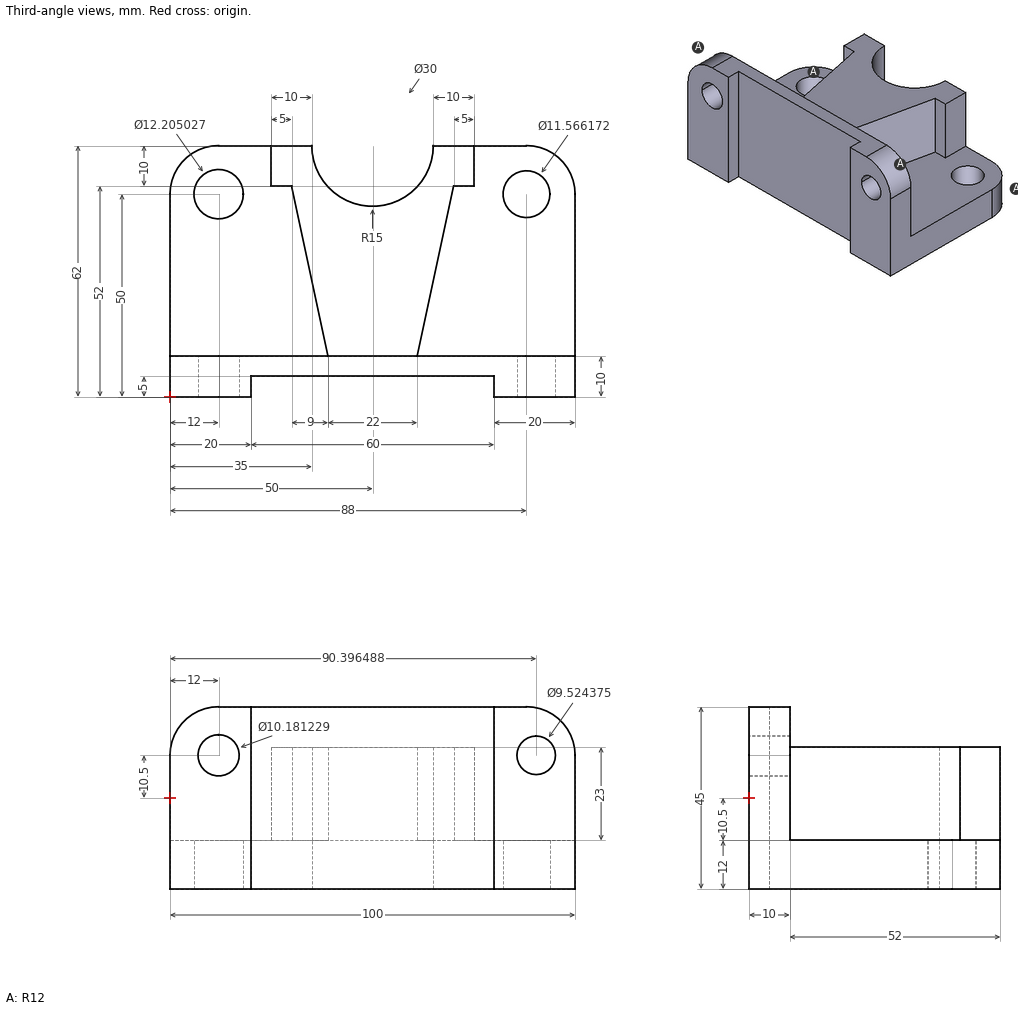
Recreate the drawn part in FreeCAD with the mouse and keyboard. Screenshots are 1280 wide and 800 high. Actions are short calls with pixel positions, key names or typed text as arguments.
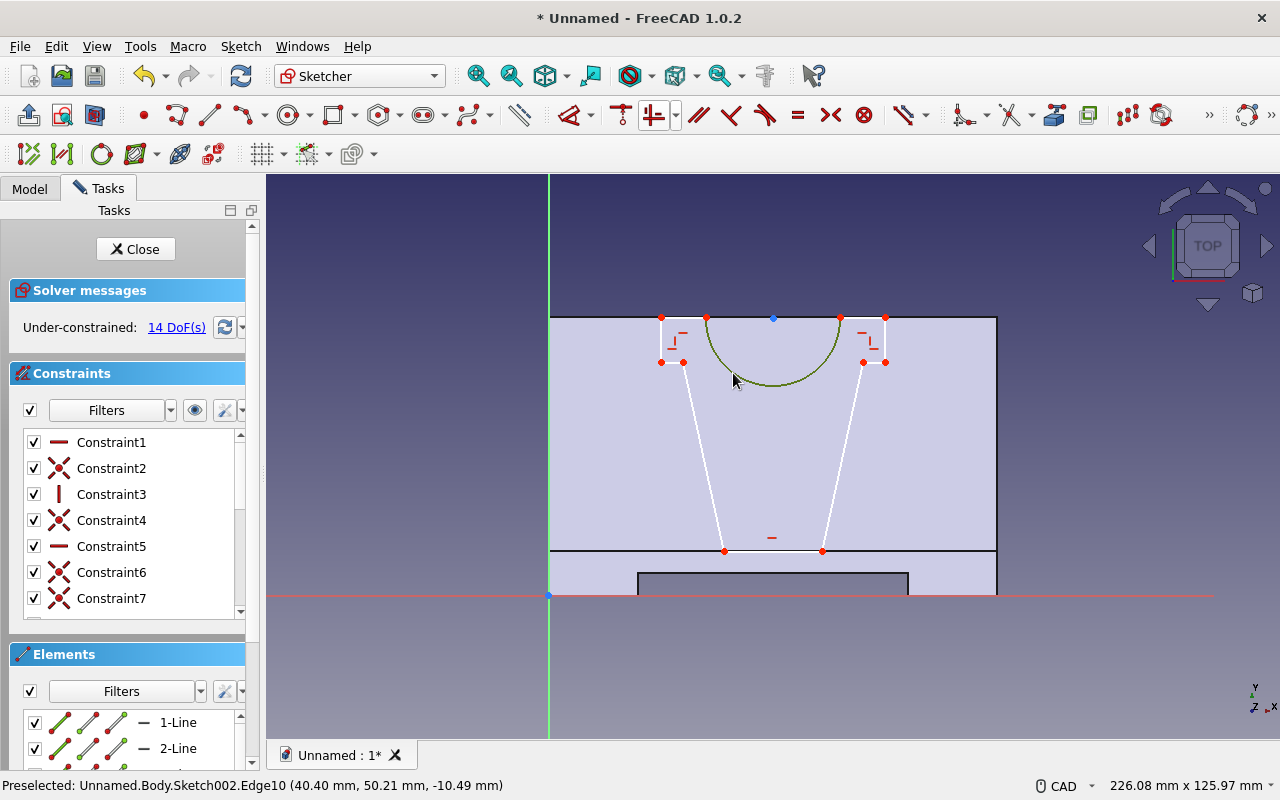
key(k)
key(r)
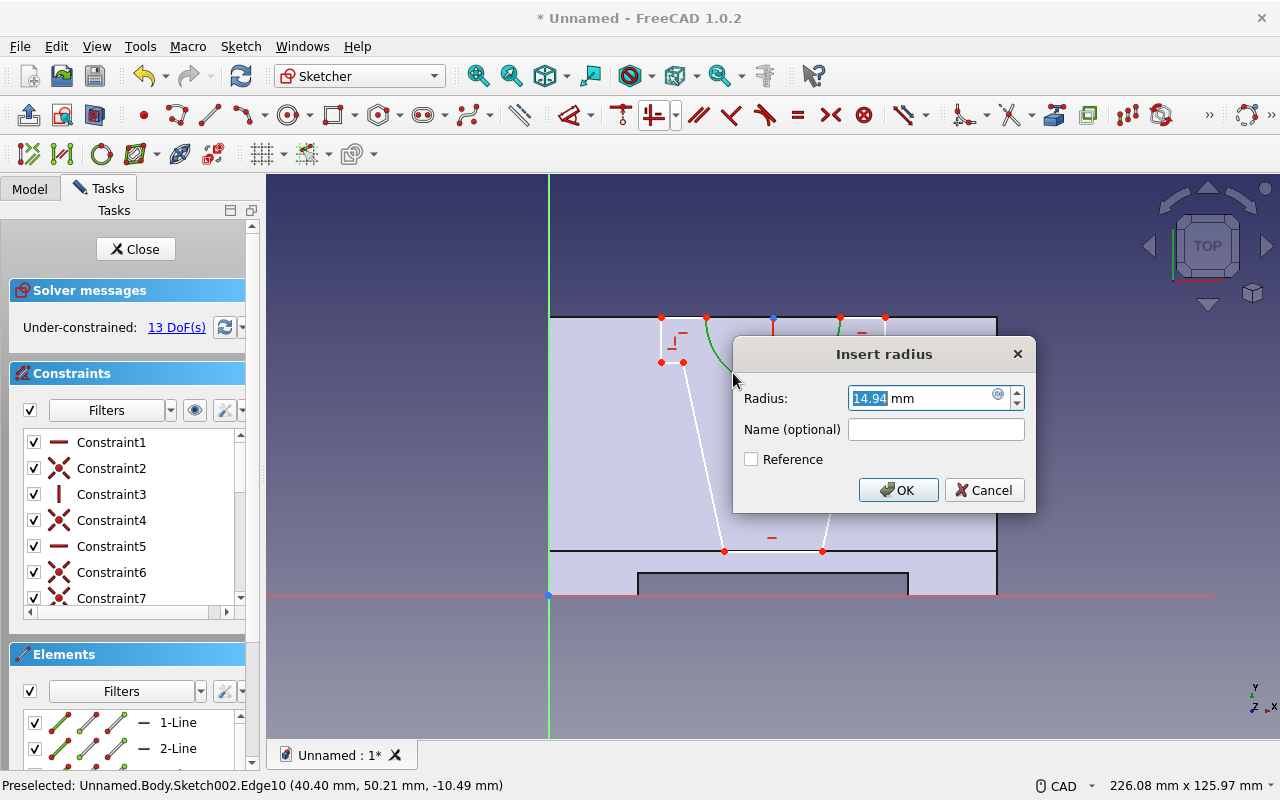
text(15)
key(Return)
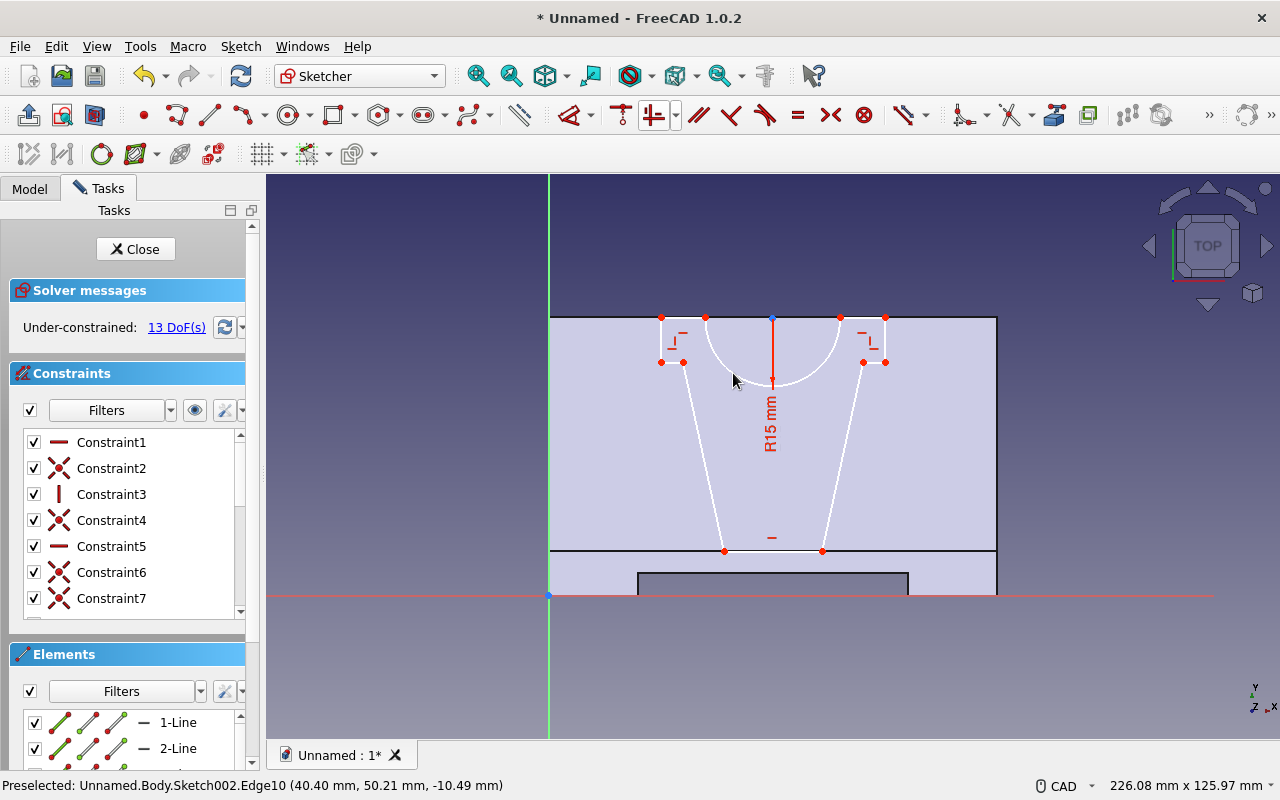
scroll(672, 363, up, 3)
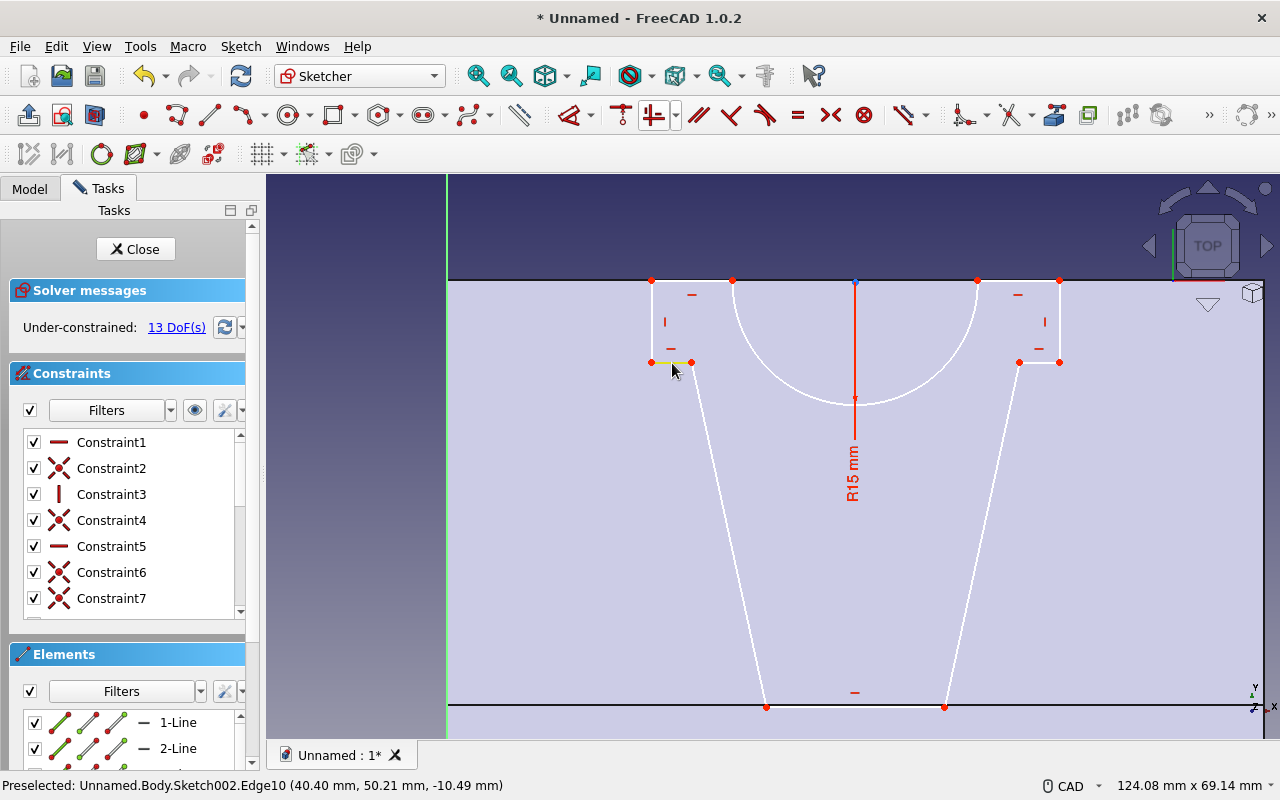
click(672, 363)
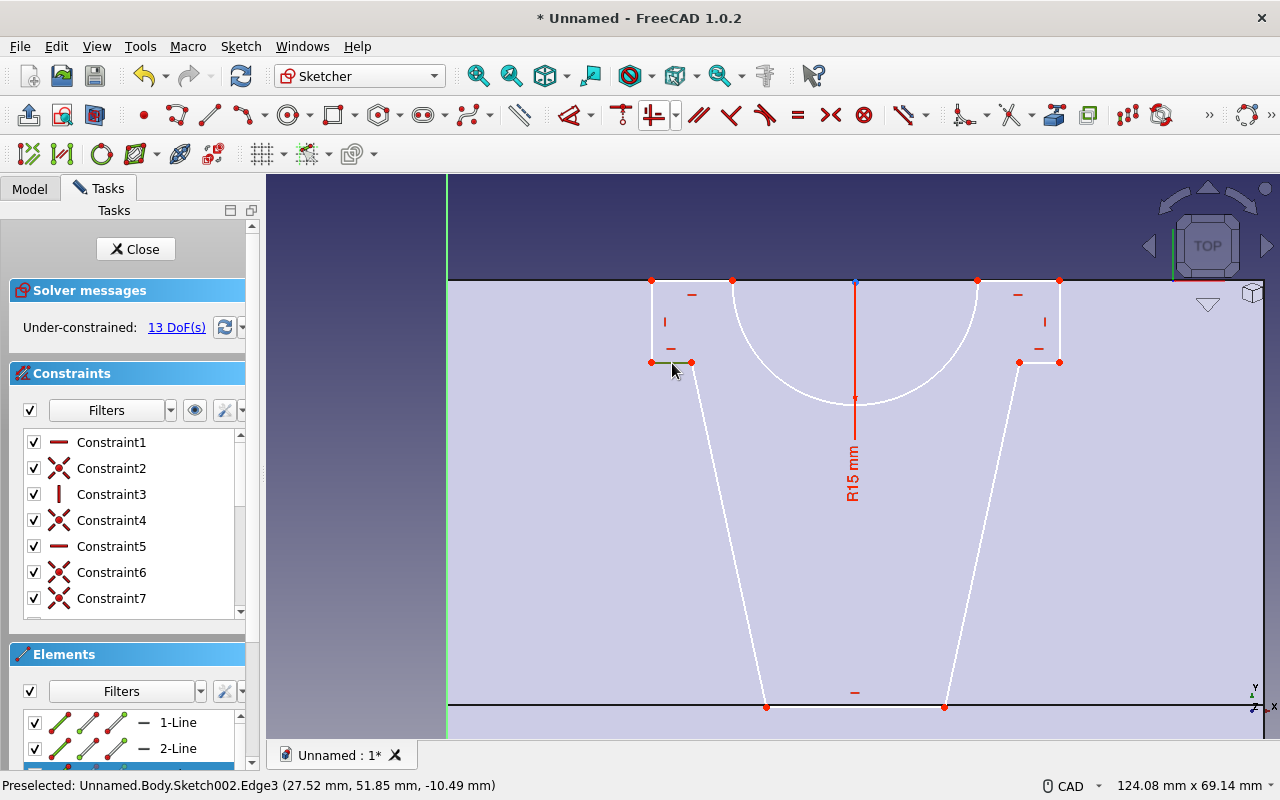
click(590, 116)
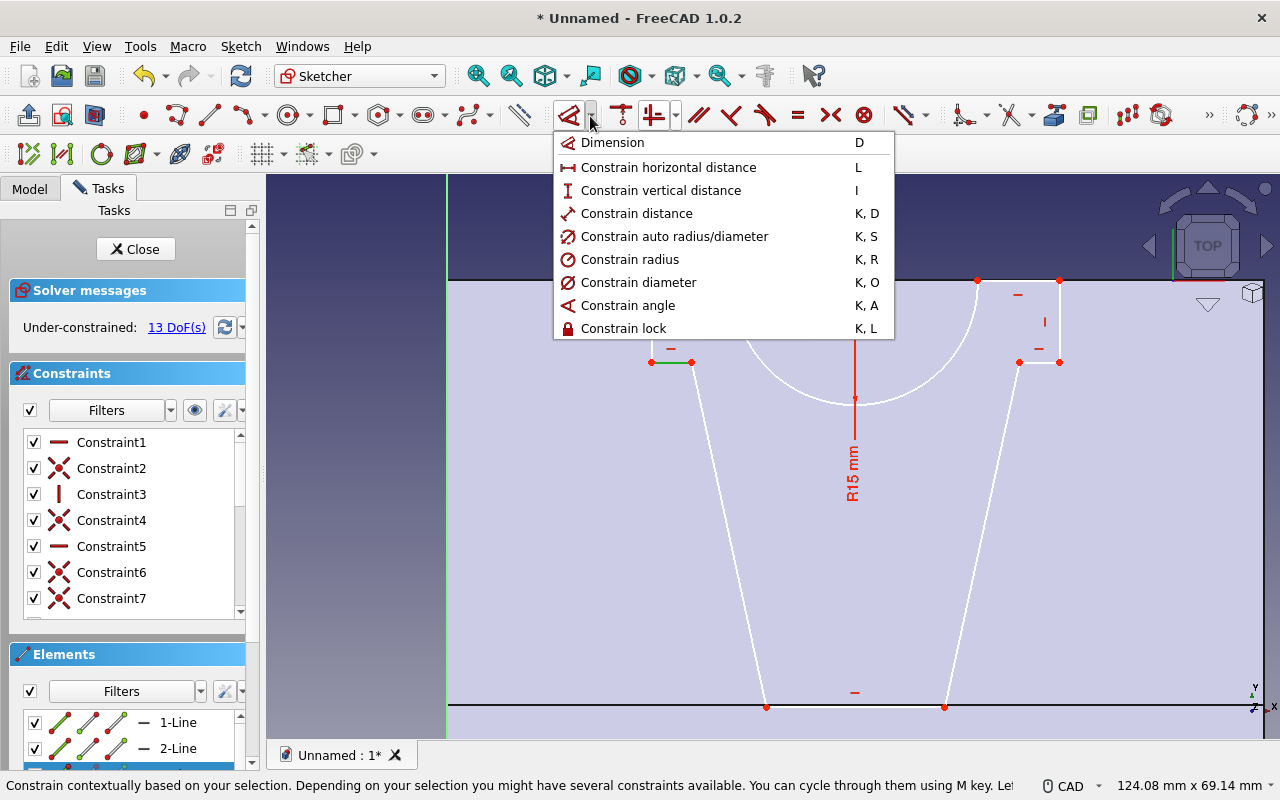
click(724, 168)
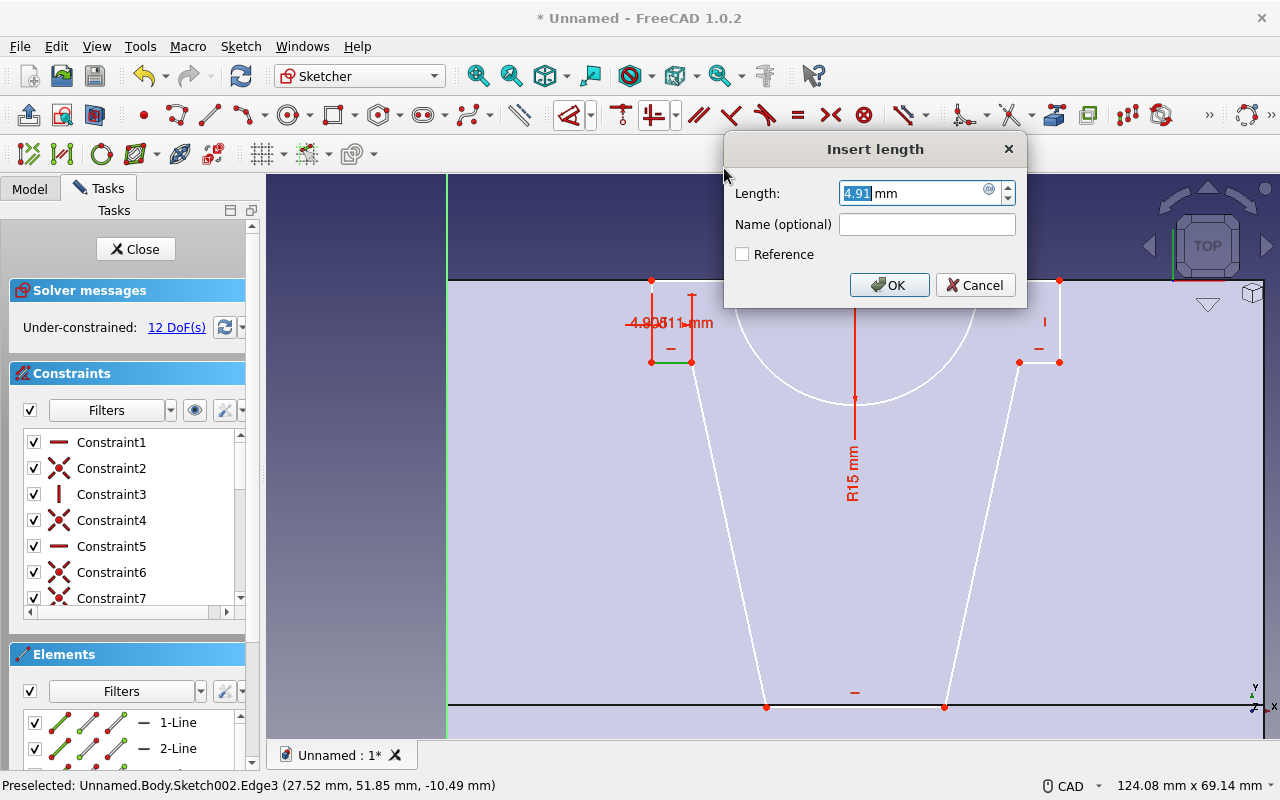
text(5)
key(Return)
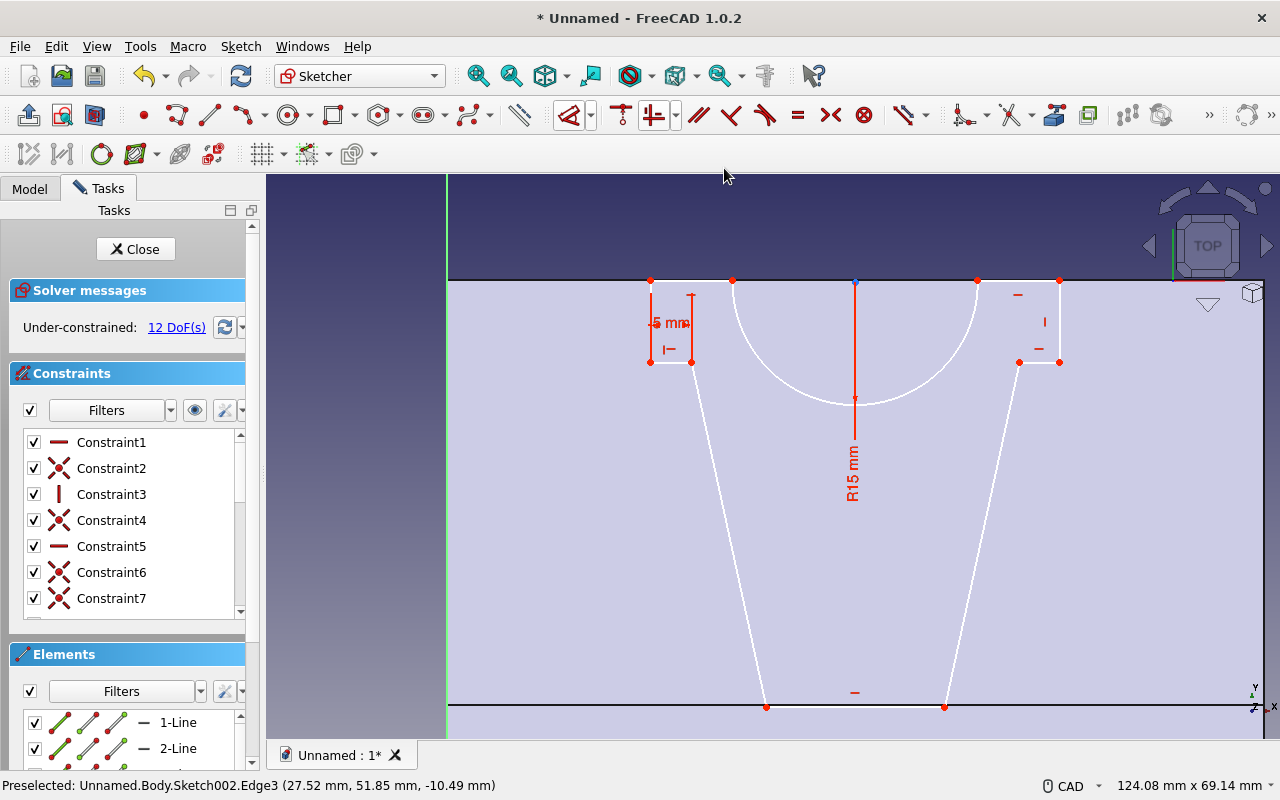
click(1032, 363)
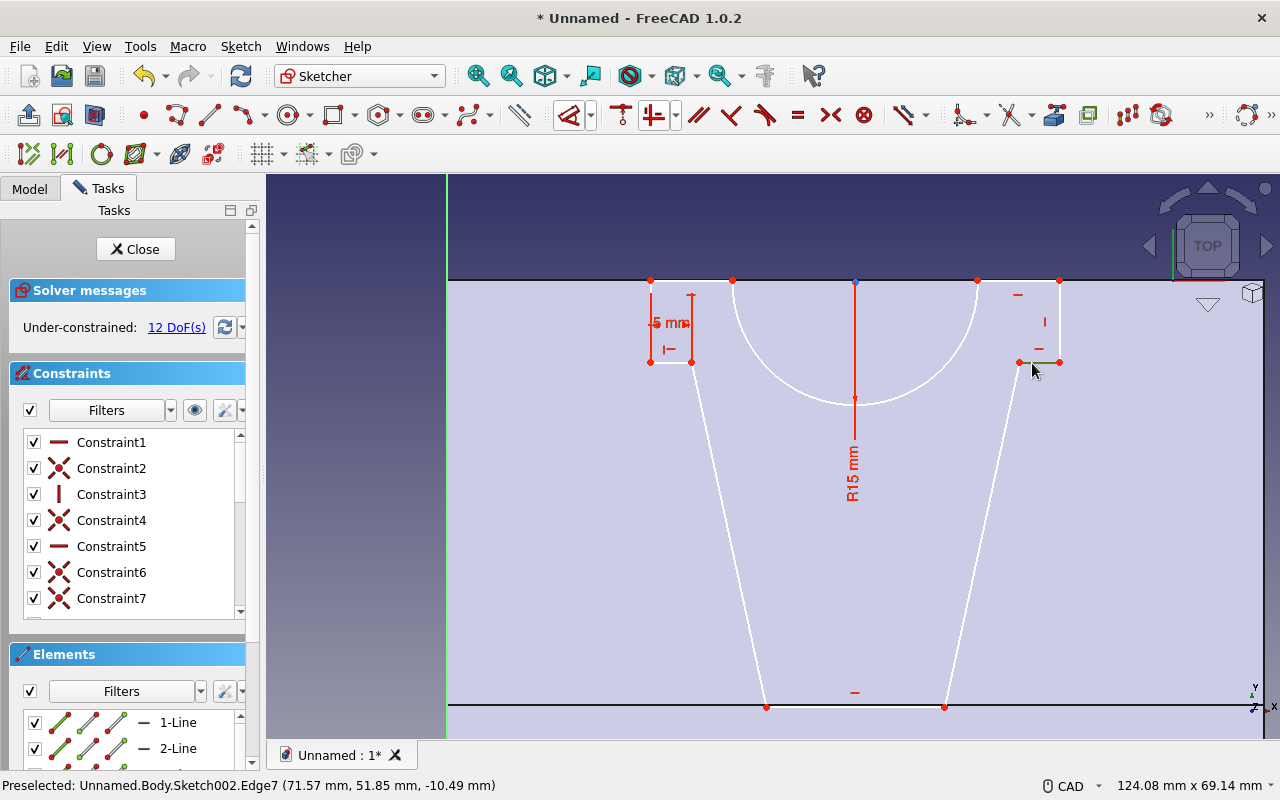
click(590, 116)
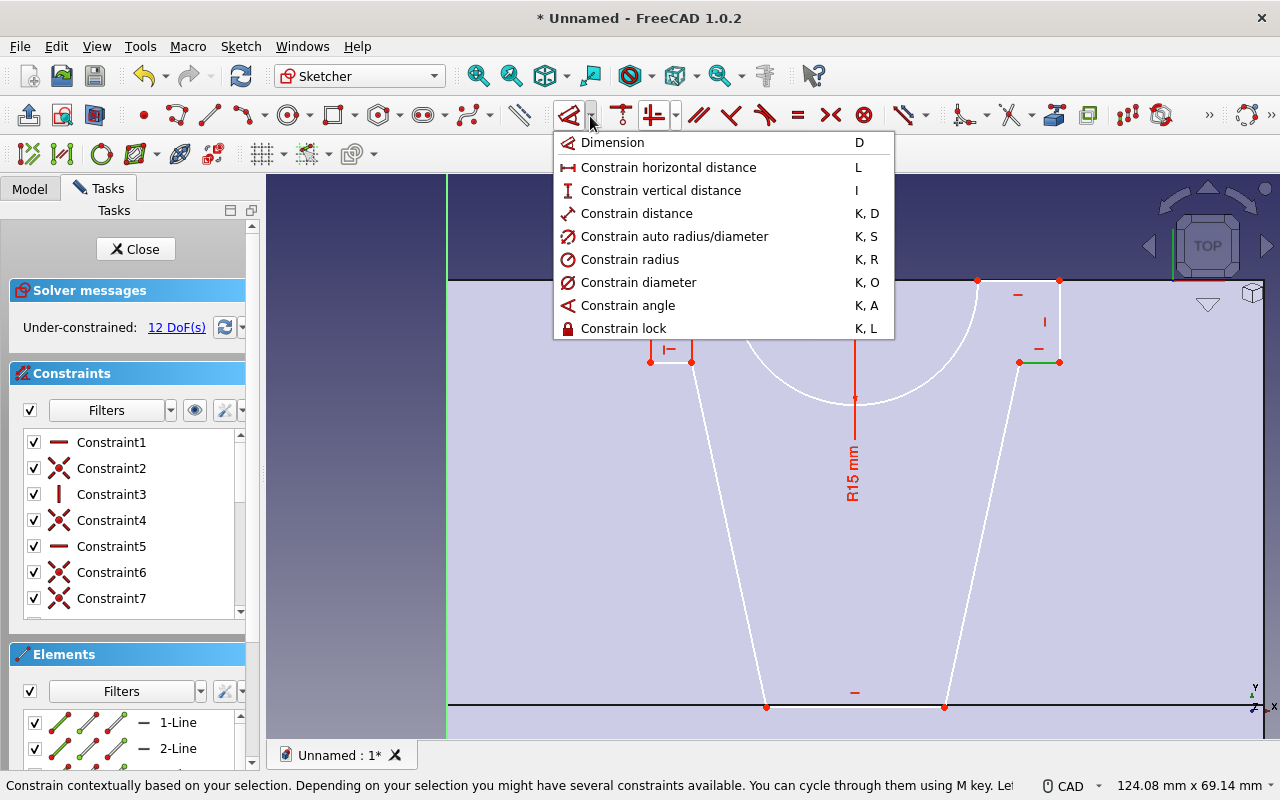
click(724, 168)